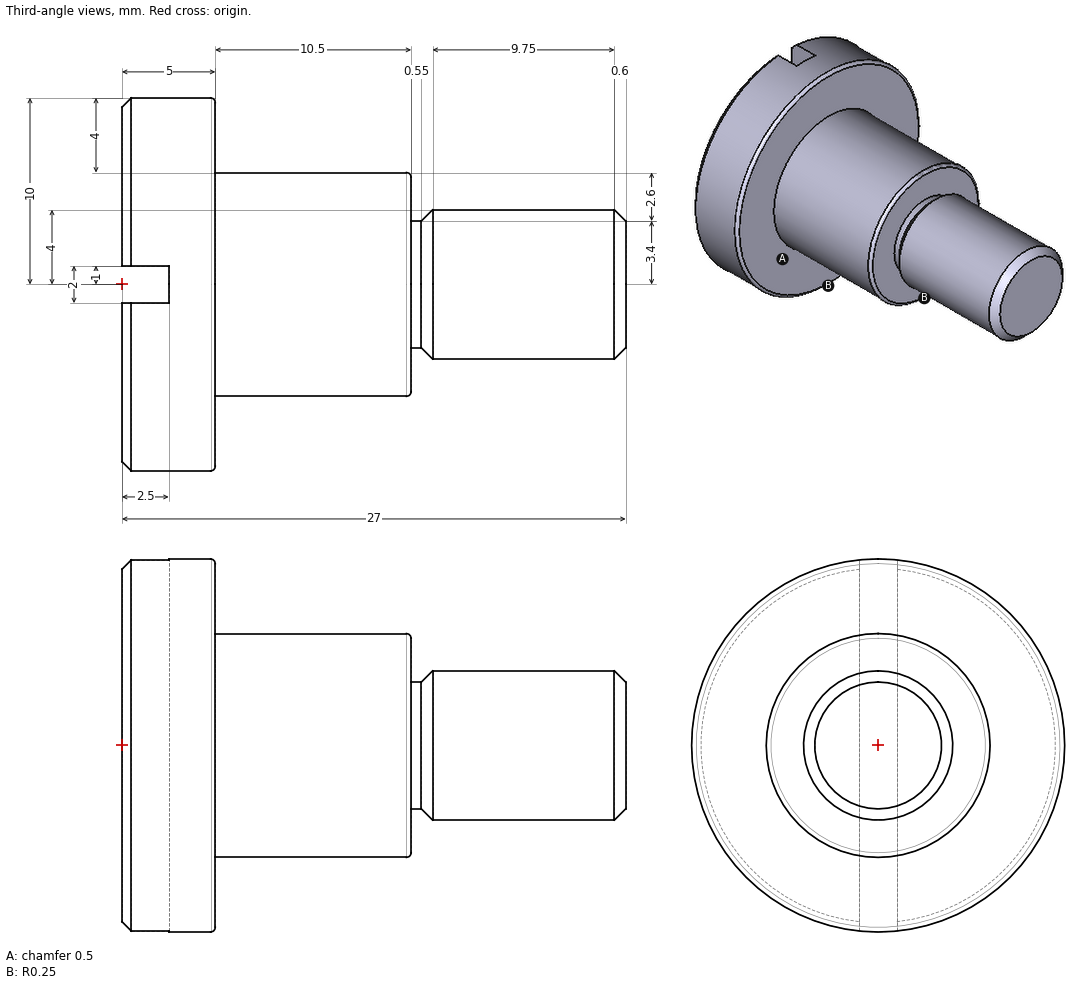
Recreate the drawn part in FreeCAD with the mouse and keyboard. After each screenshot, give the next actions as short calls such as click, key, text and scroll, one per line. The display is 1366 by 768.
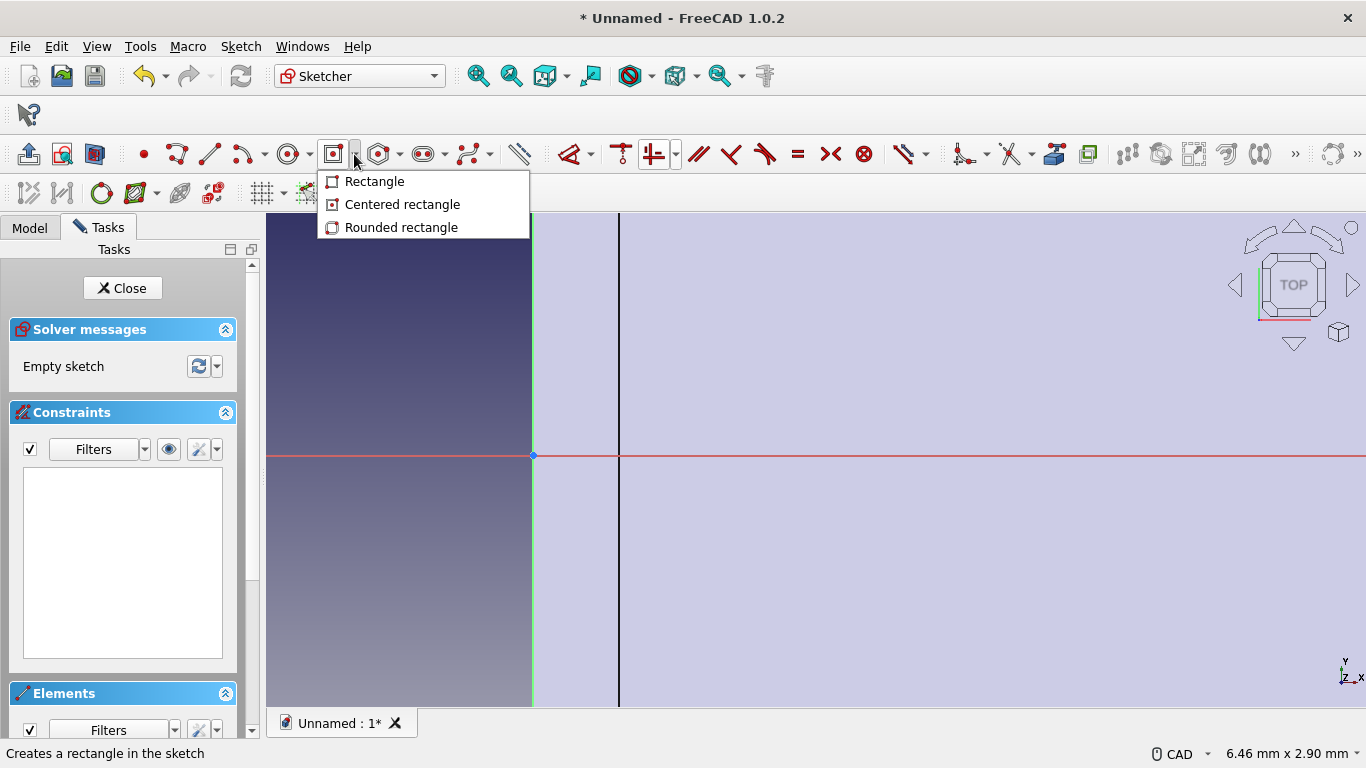
click(424, 182)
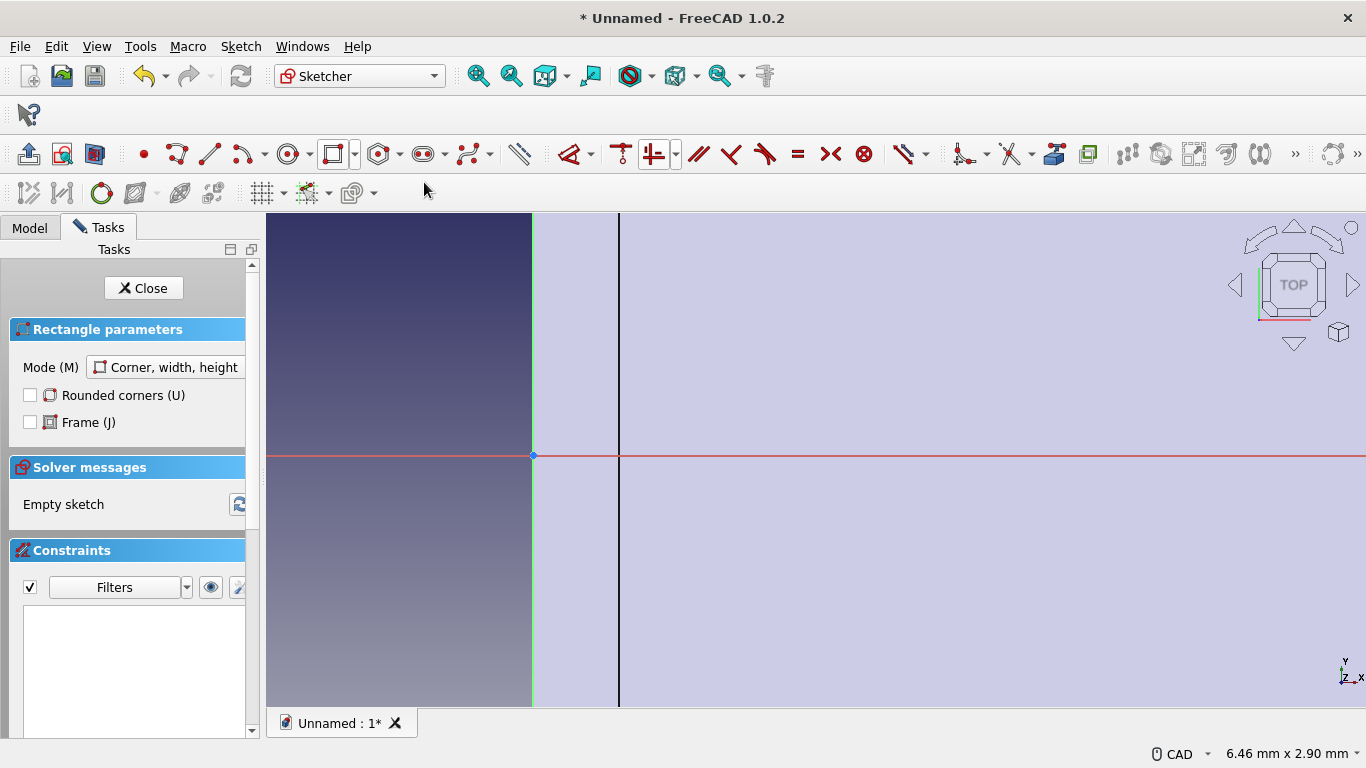
click(533, 285)
move(959, 626)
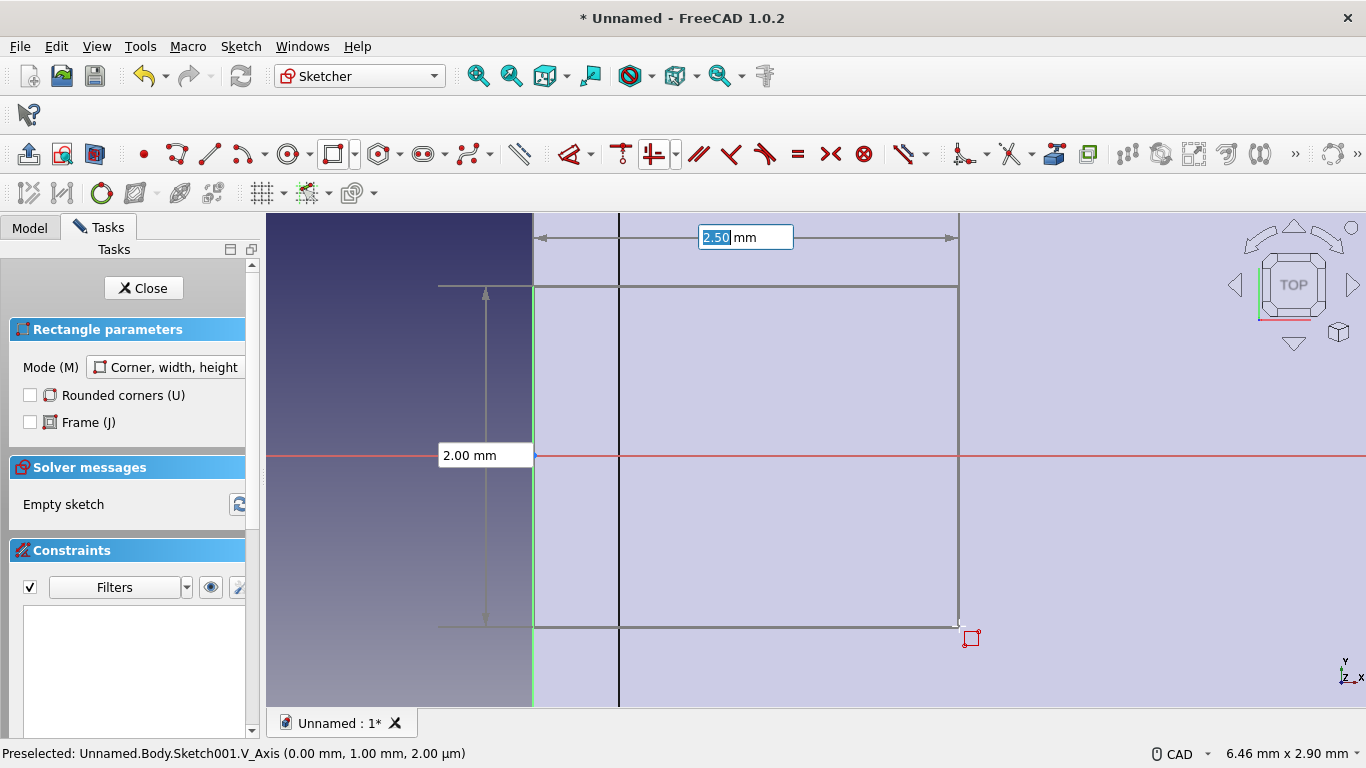
text(2.5)
key(Tab)
text(2)
key(Return)
key(Escape)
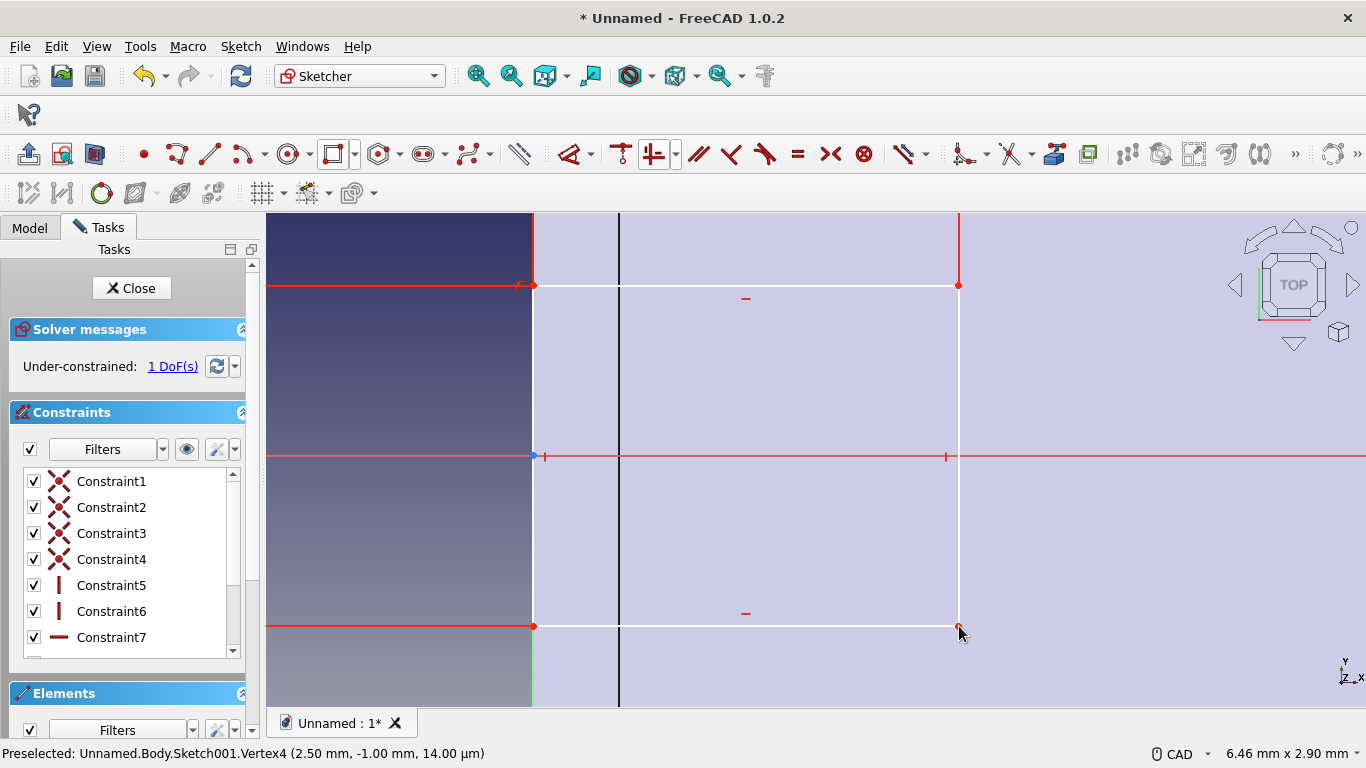
click(568, 154)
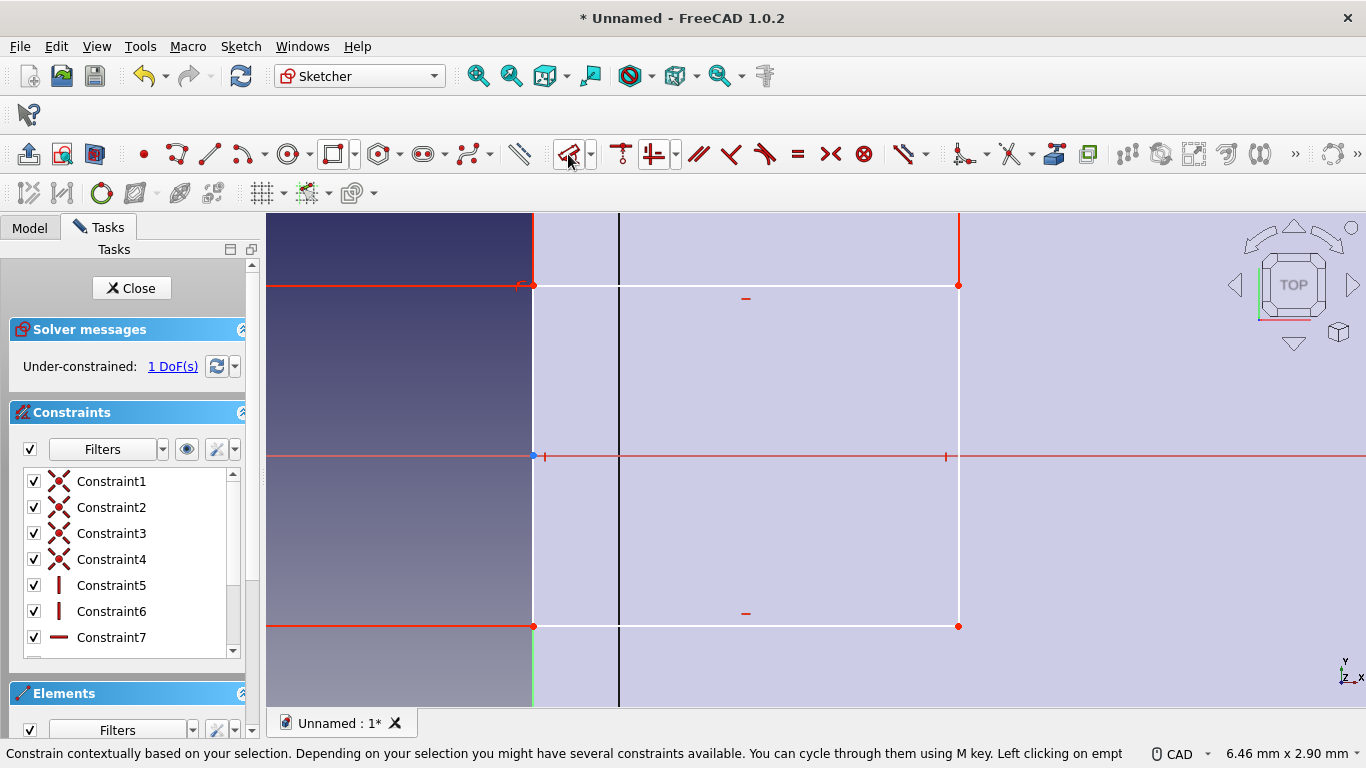
click(533, 286)
click(499, 371)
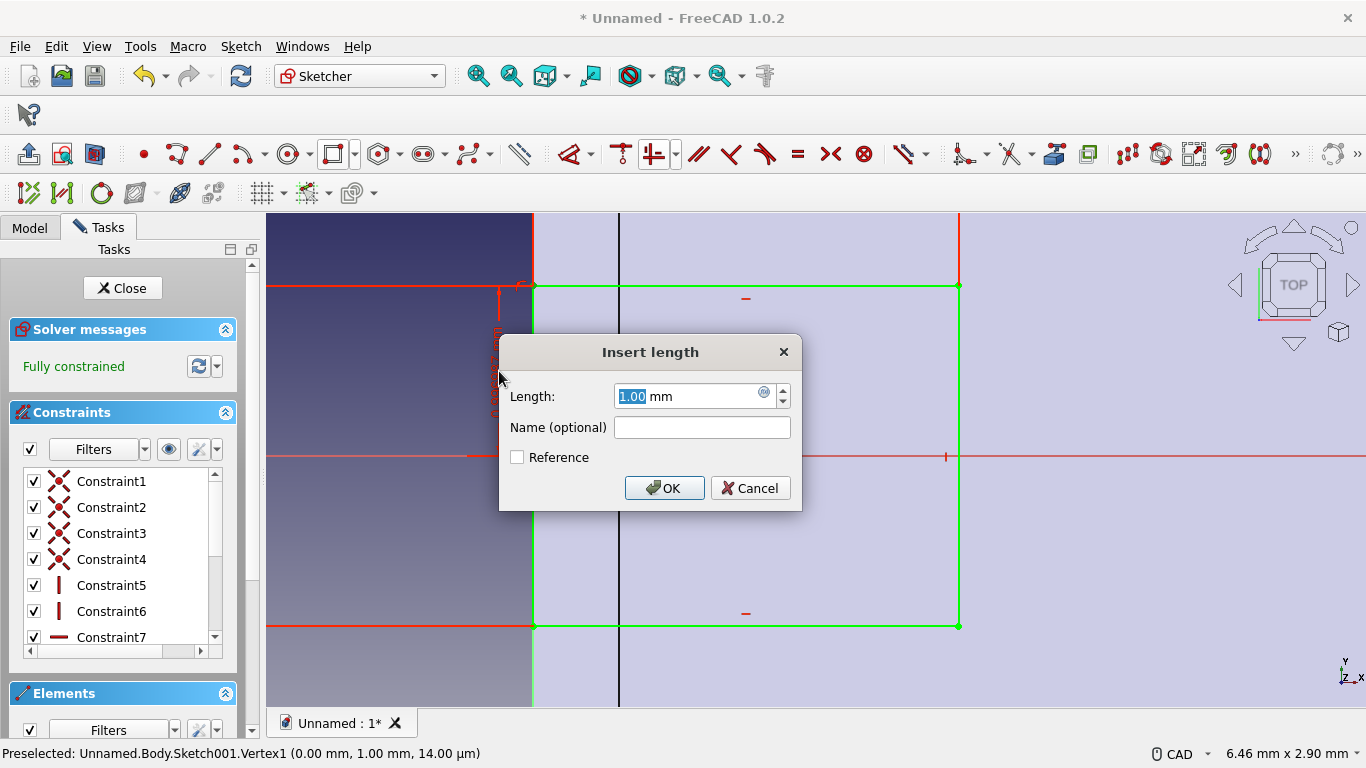
text(1)
key(Return)
key(Escape)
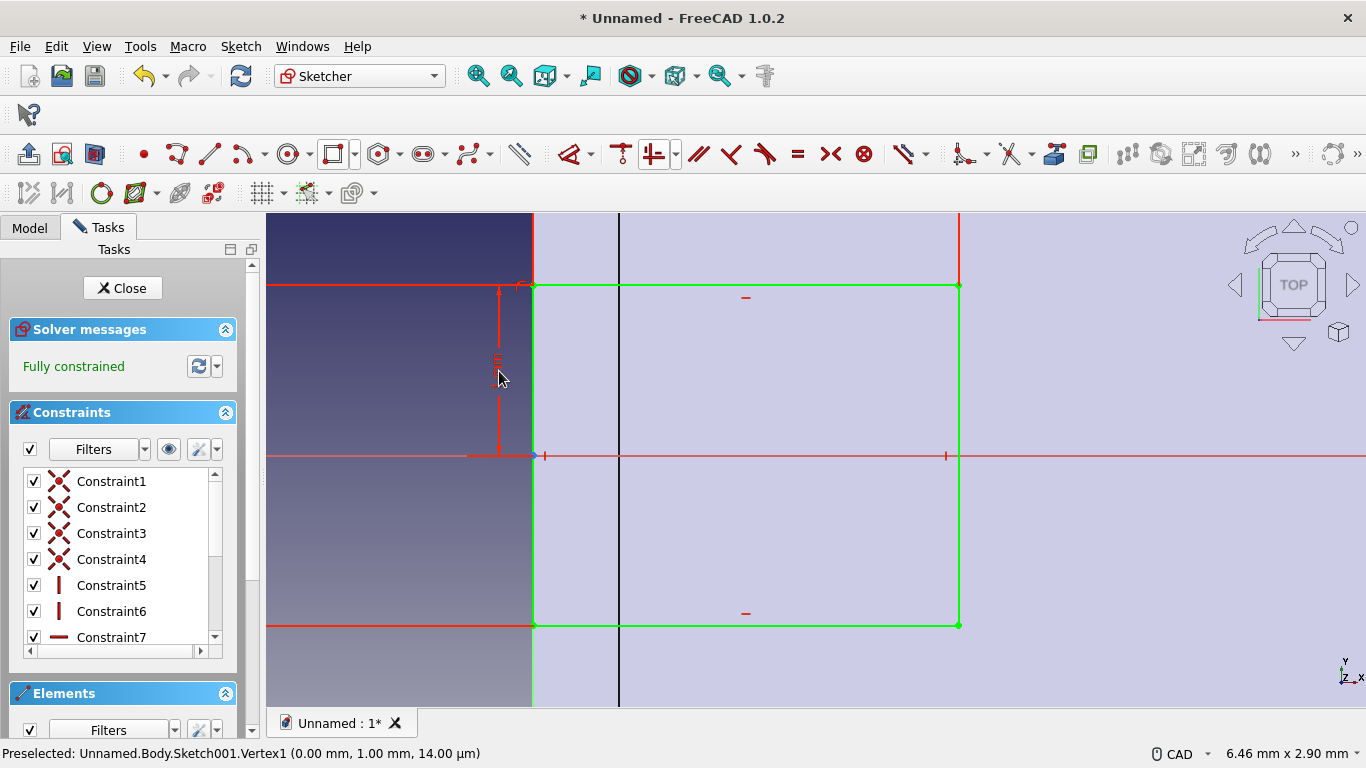
click(123, 288)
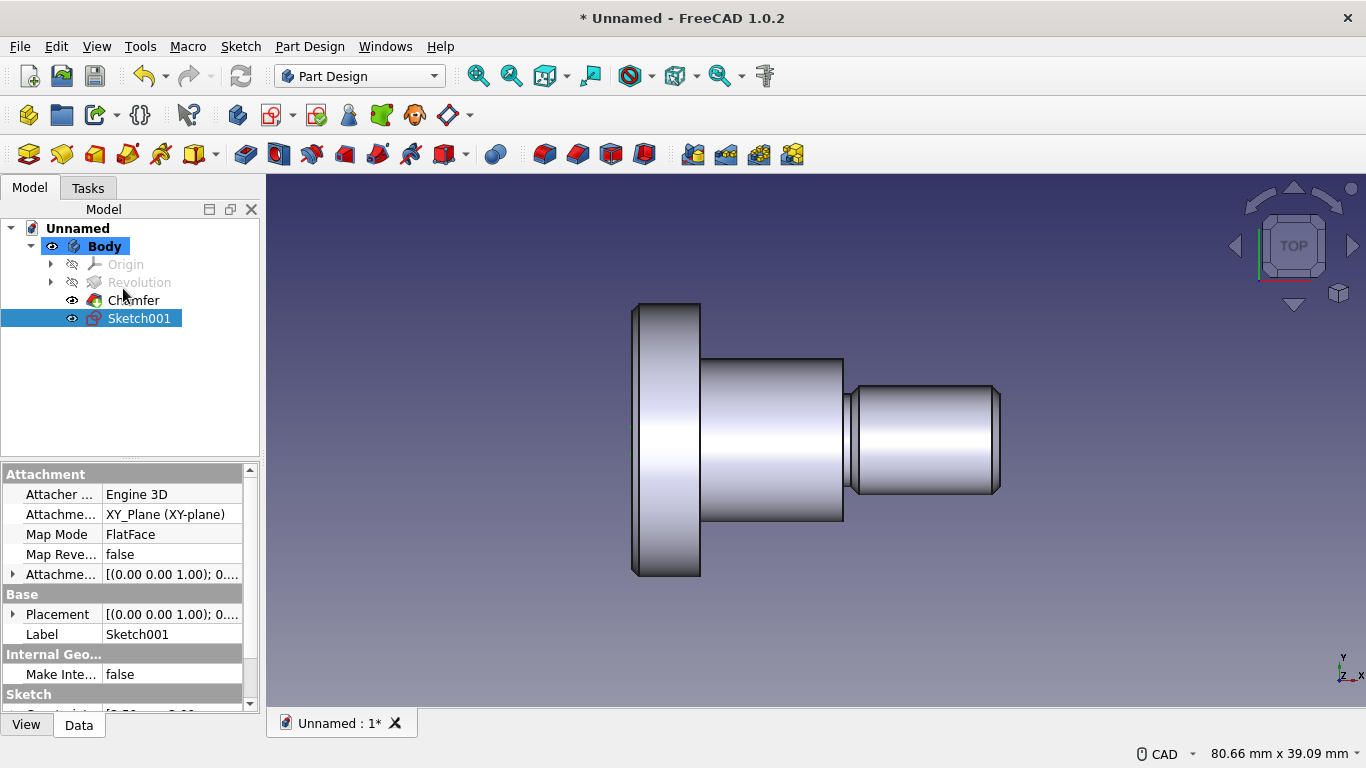
click(246, 154)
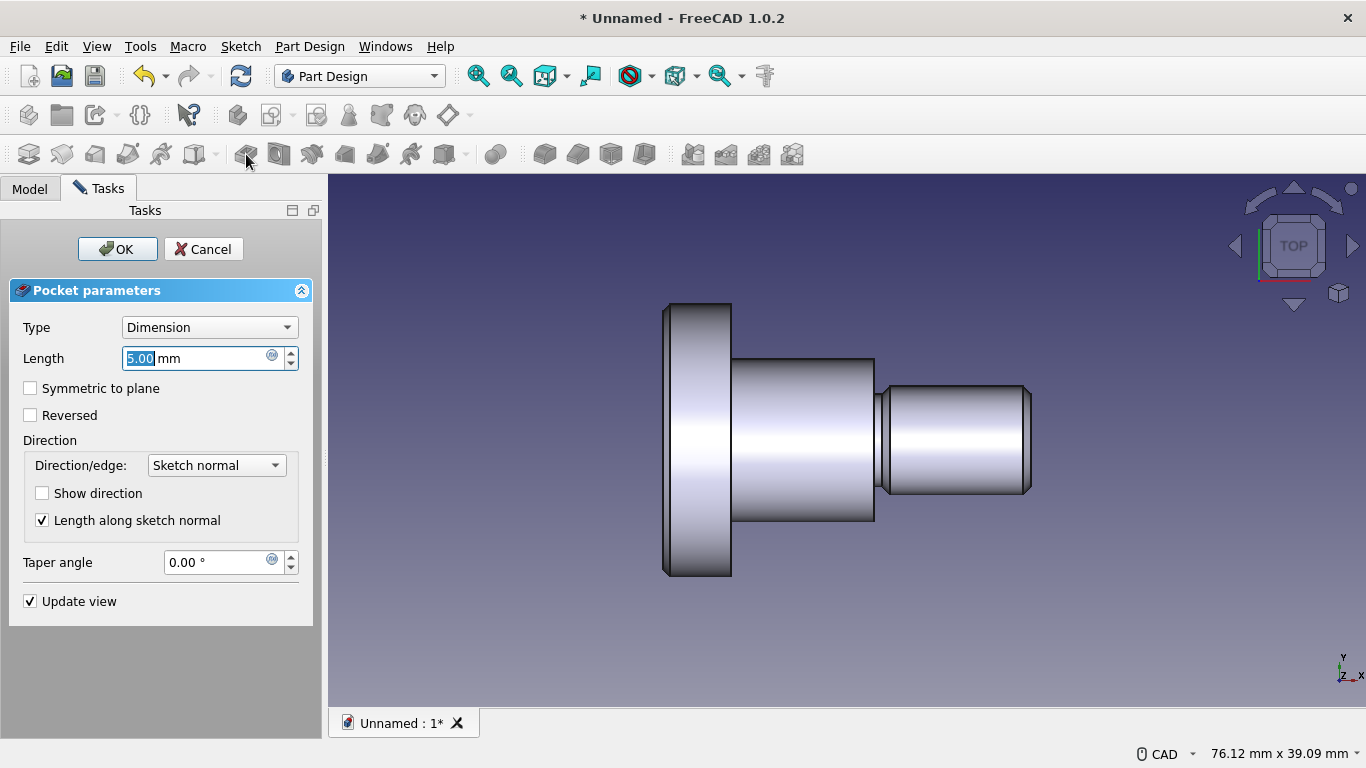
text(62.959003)
key(Tab)